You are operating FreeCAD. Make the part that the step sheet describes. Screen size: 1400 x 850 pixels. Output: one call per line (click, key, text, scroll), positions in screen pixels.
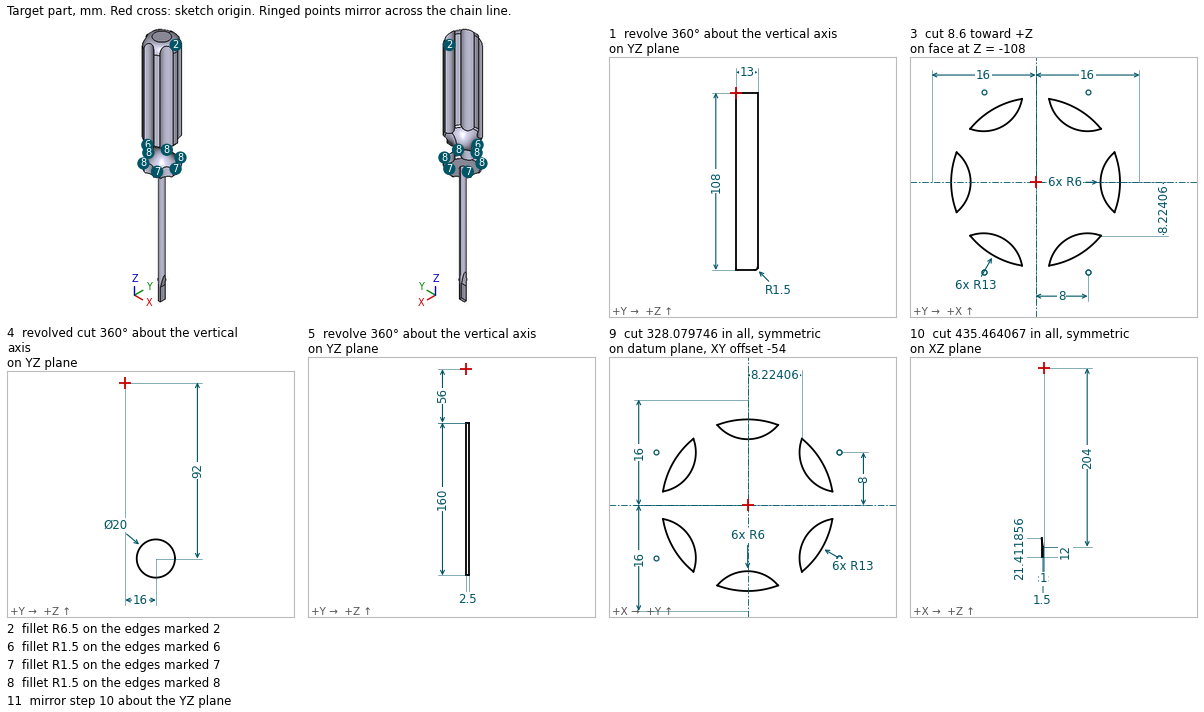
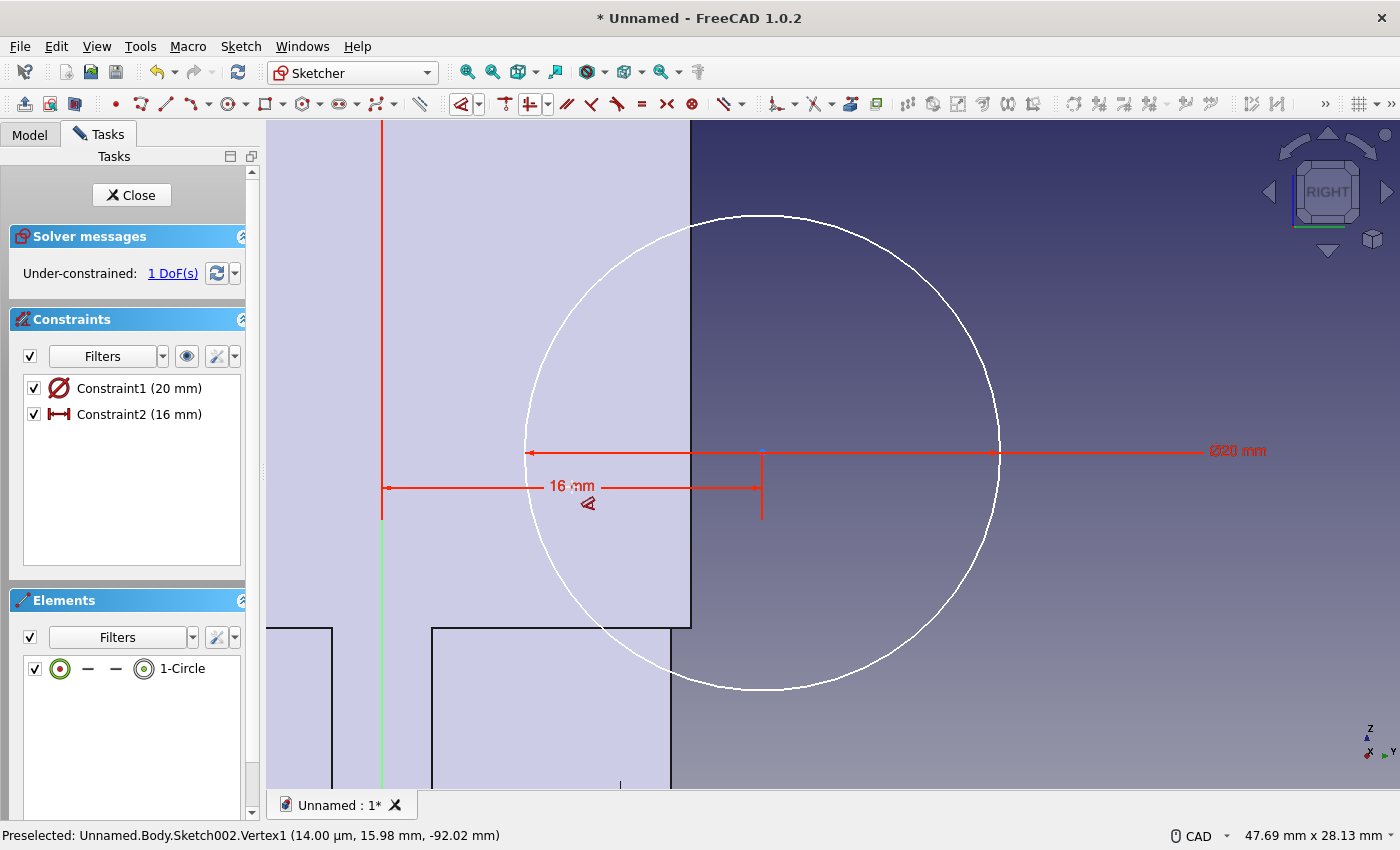
click(762, 453)
click(348, 300)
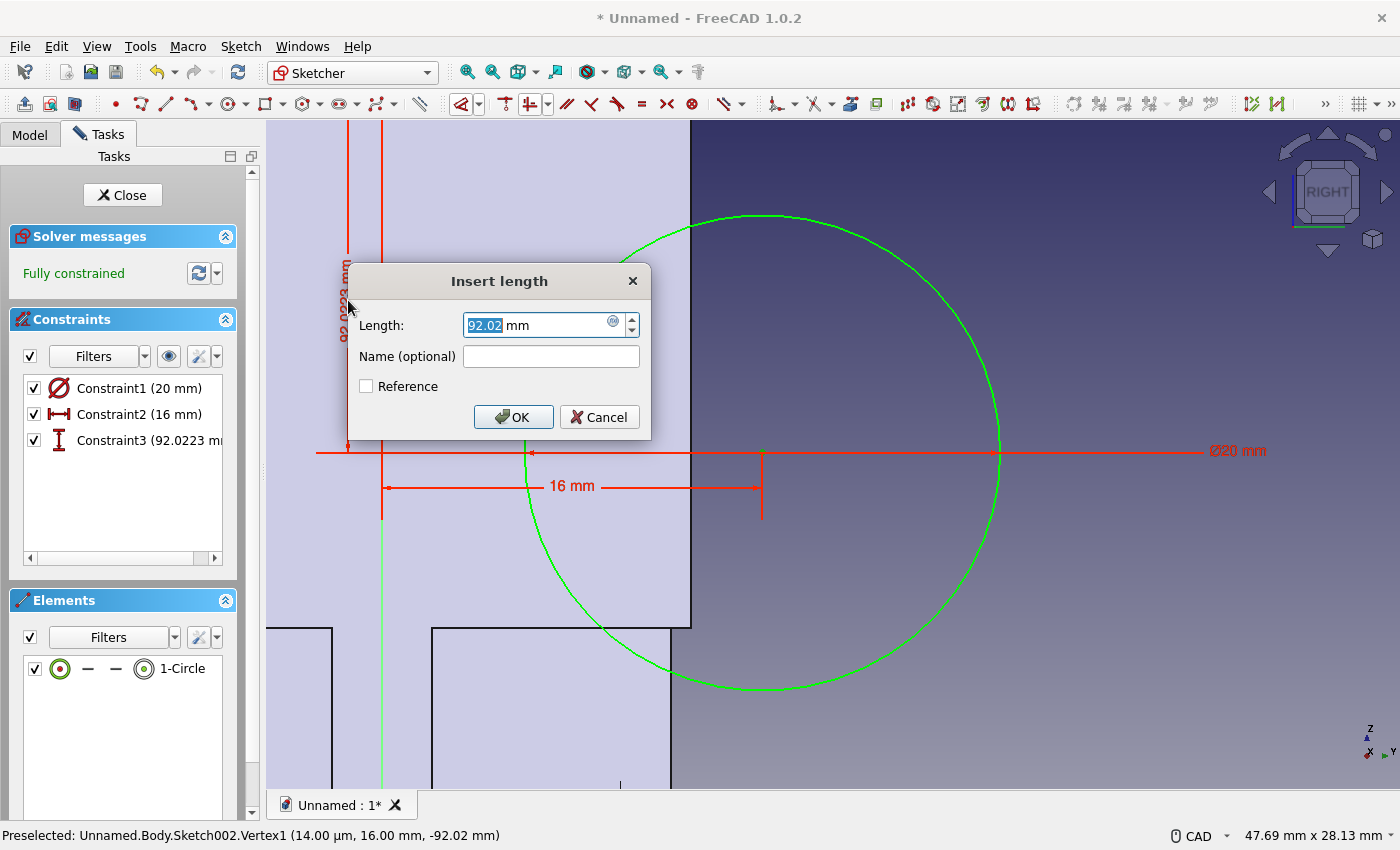
text(92)
key(Return)
key(Escape)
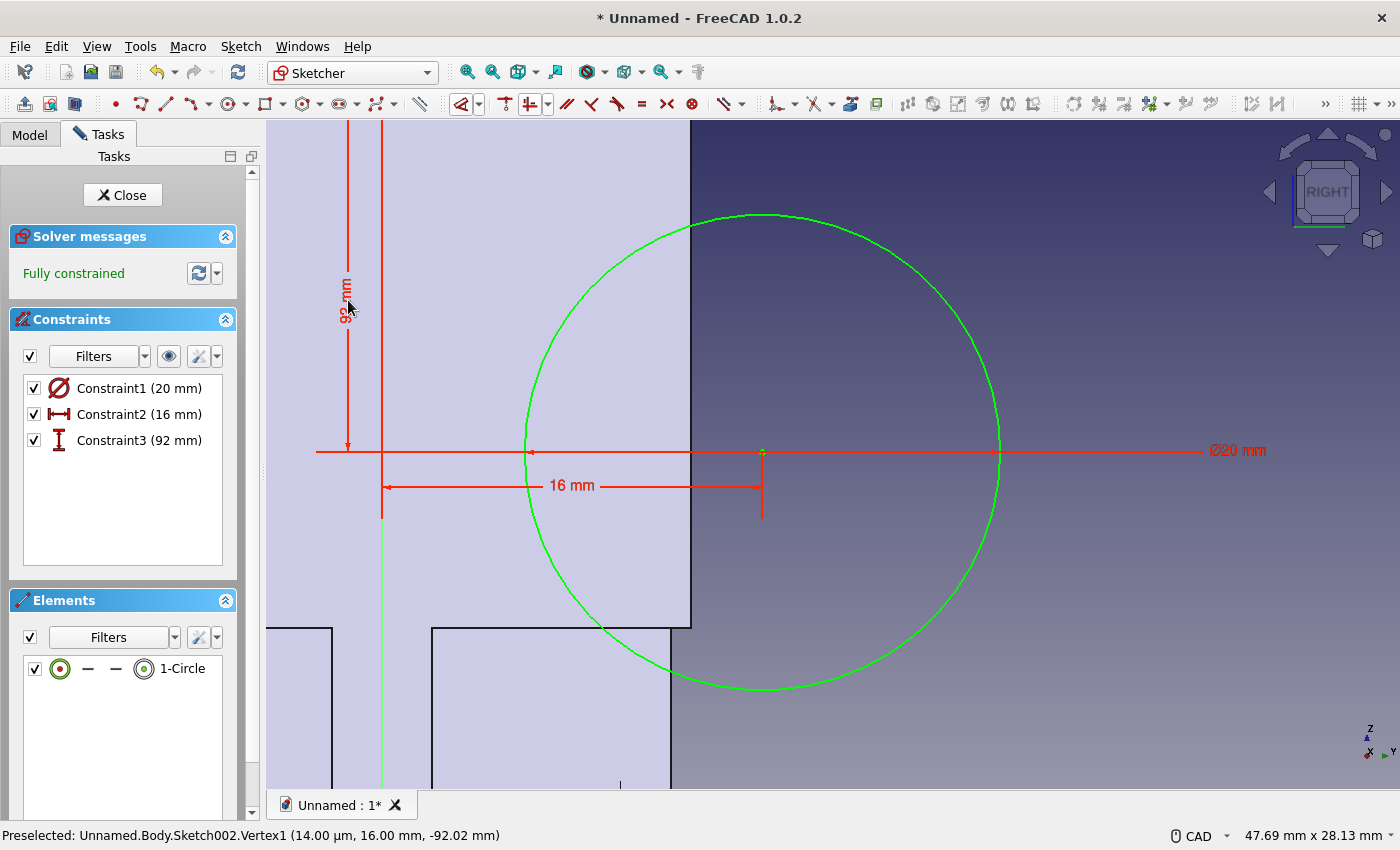
click(123, 195)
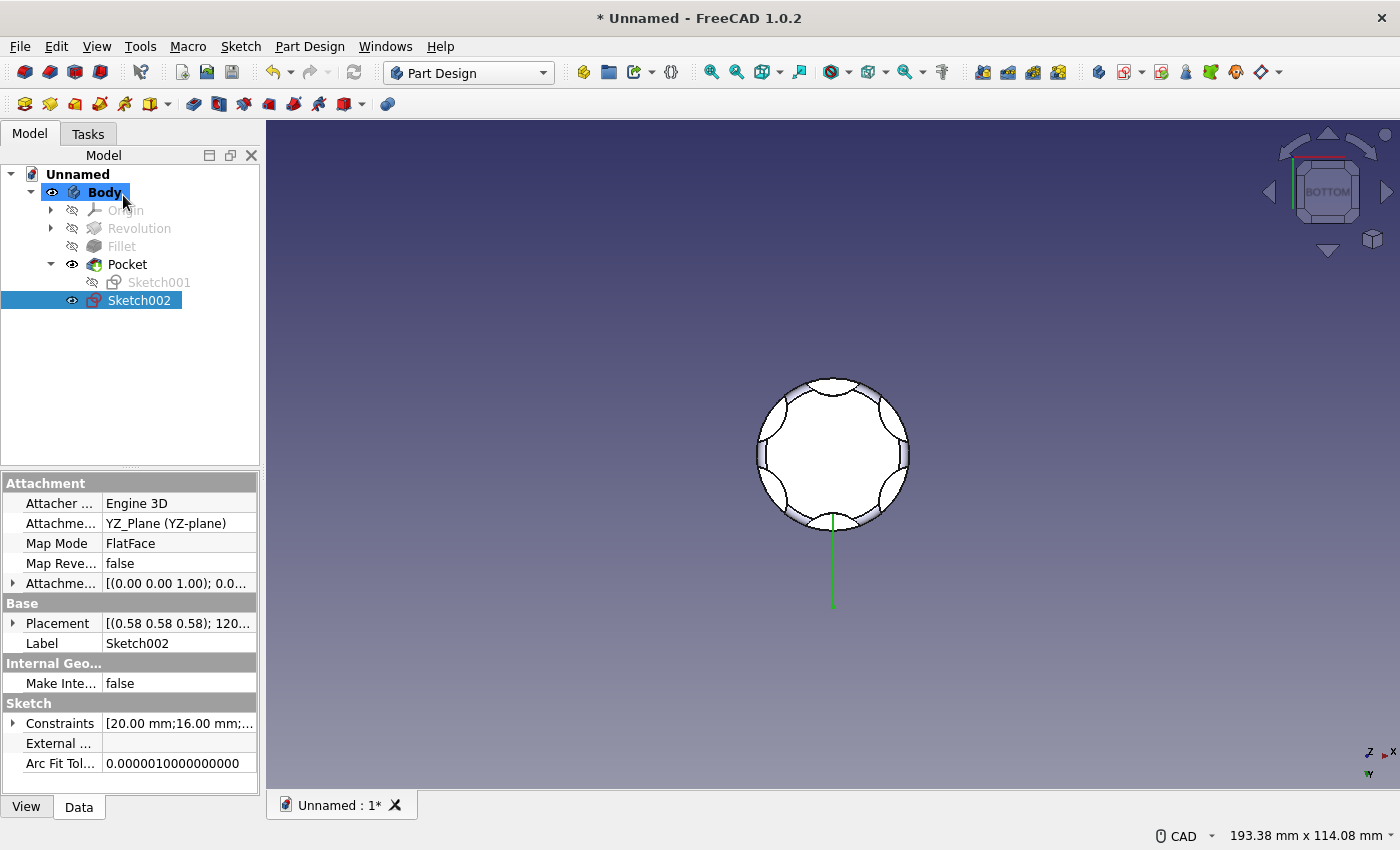
click(244, 104)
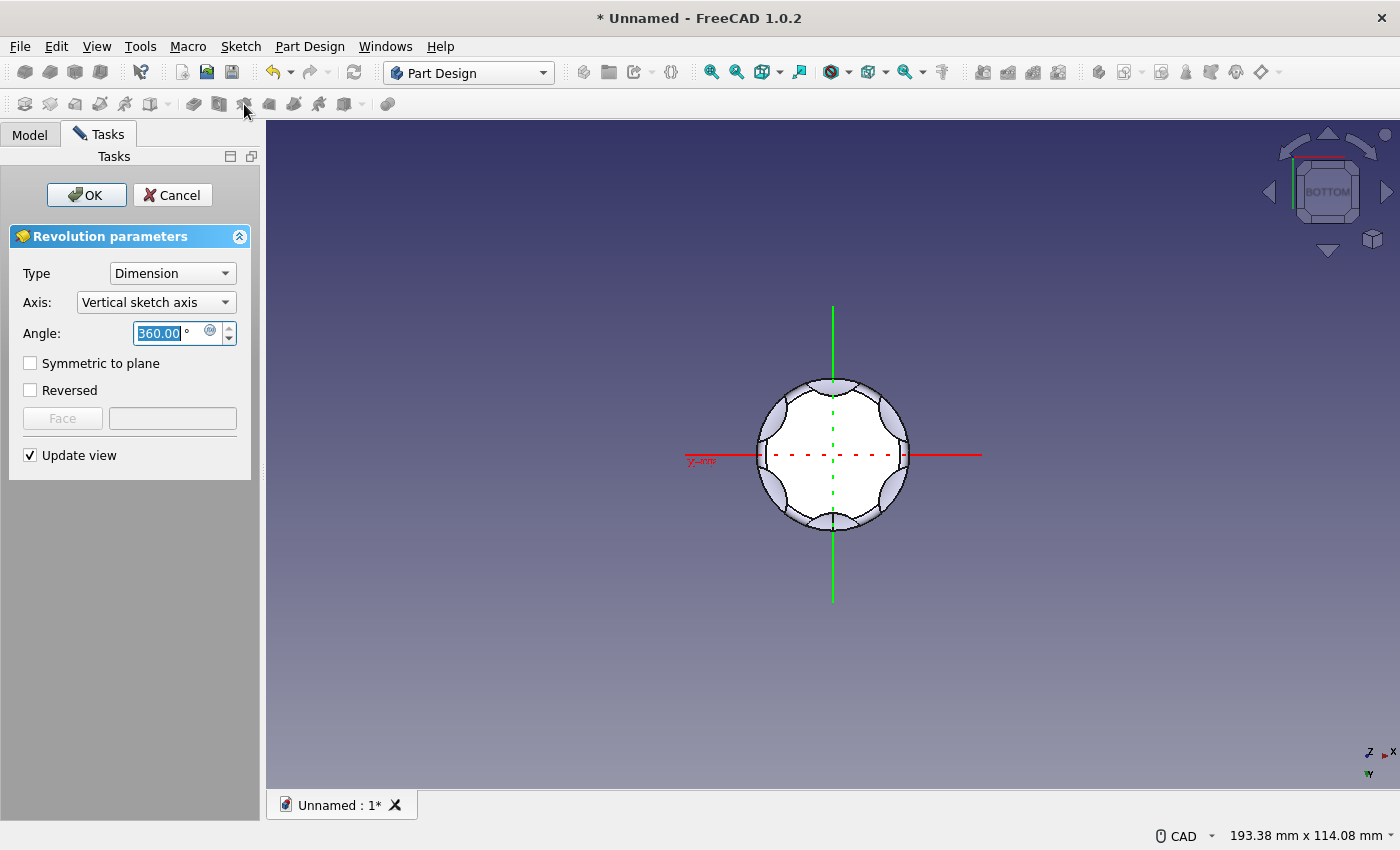
click(87, 195)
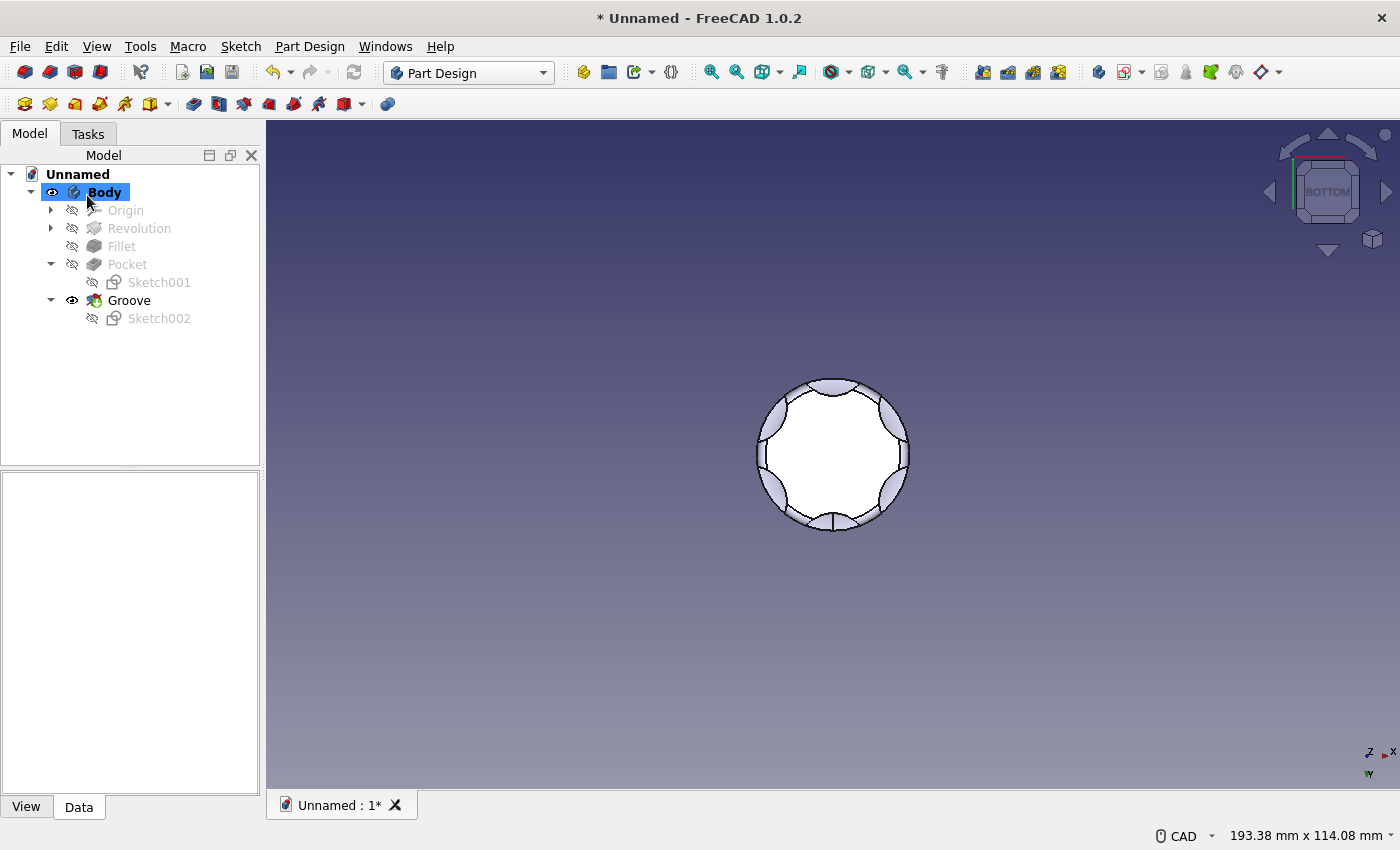
click(712, 72)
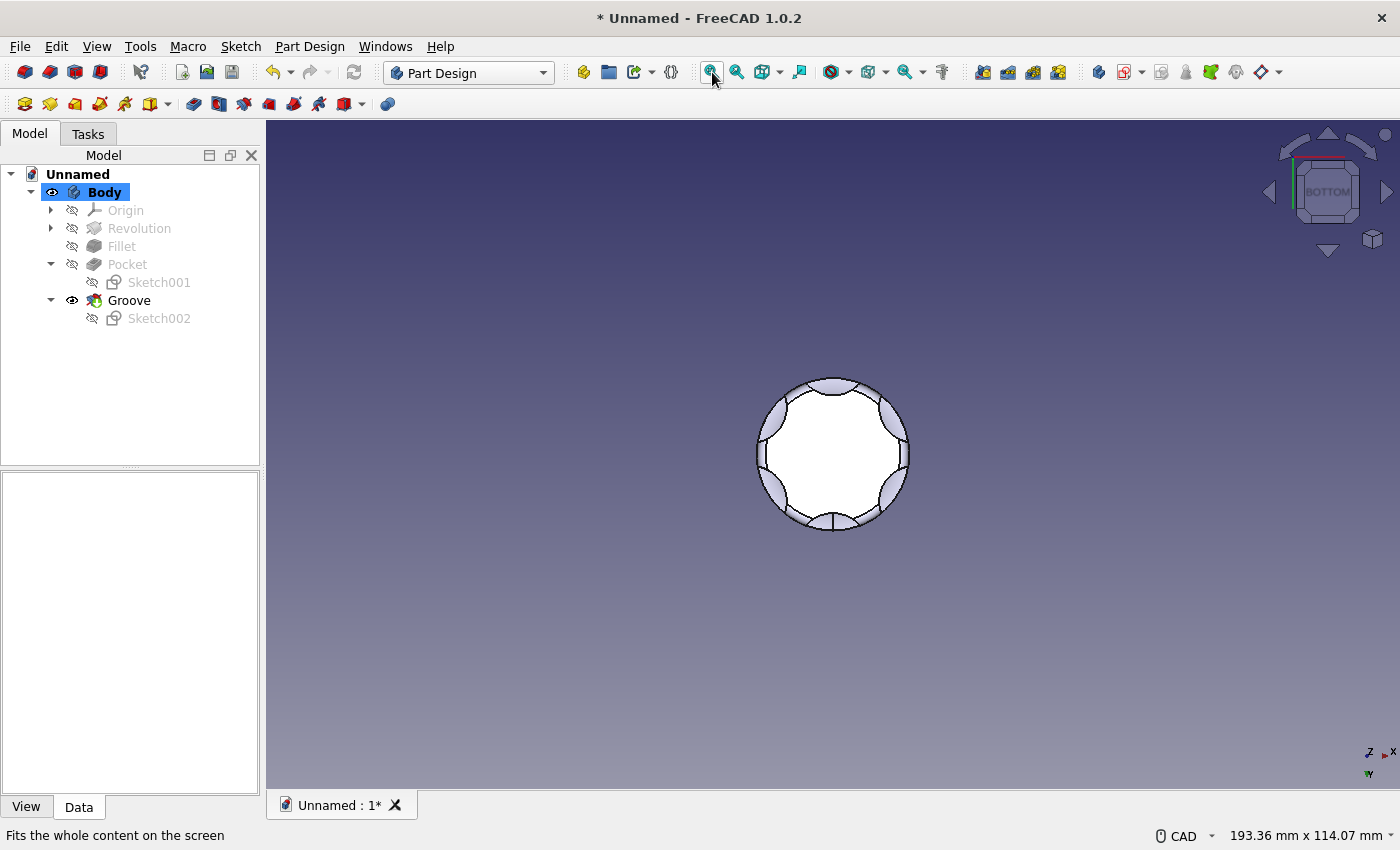
click(1124, 72)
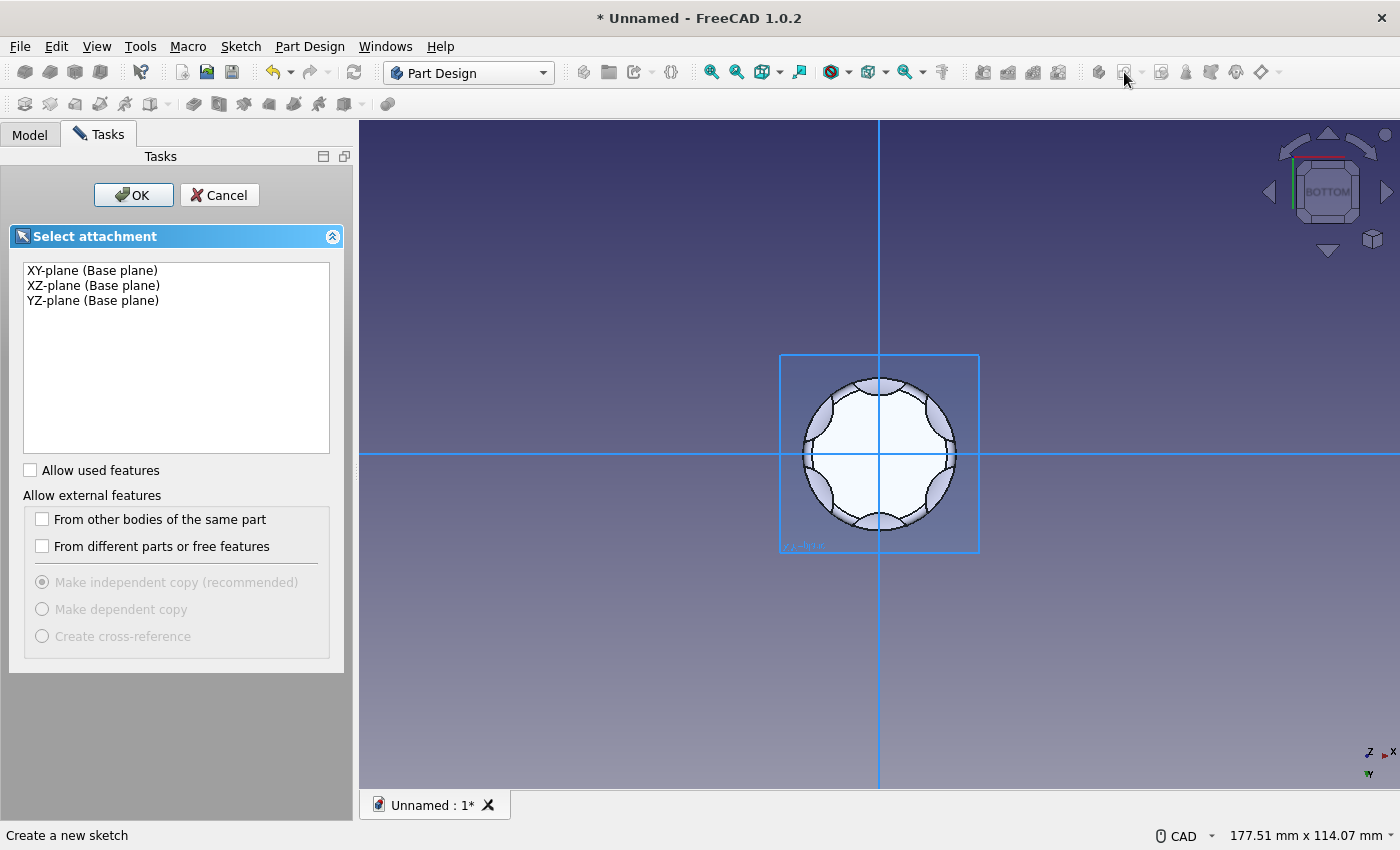
click(84, 300)